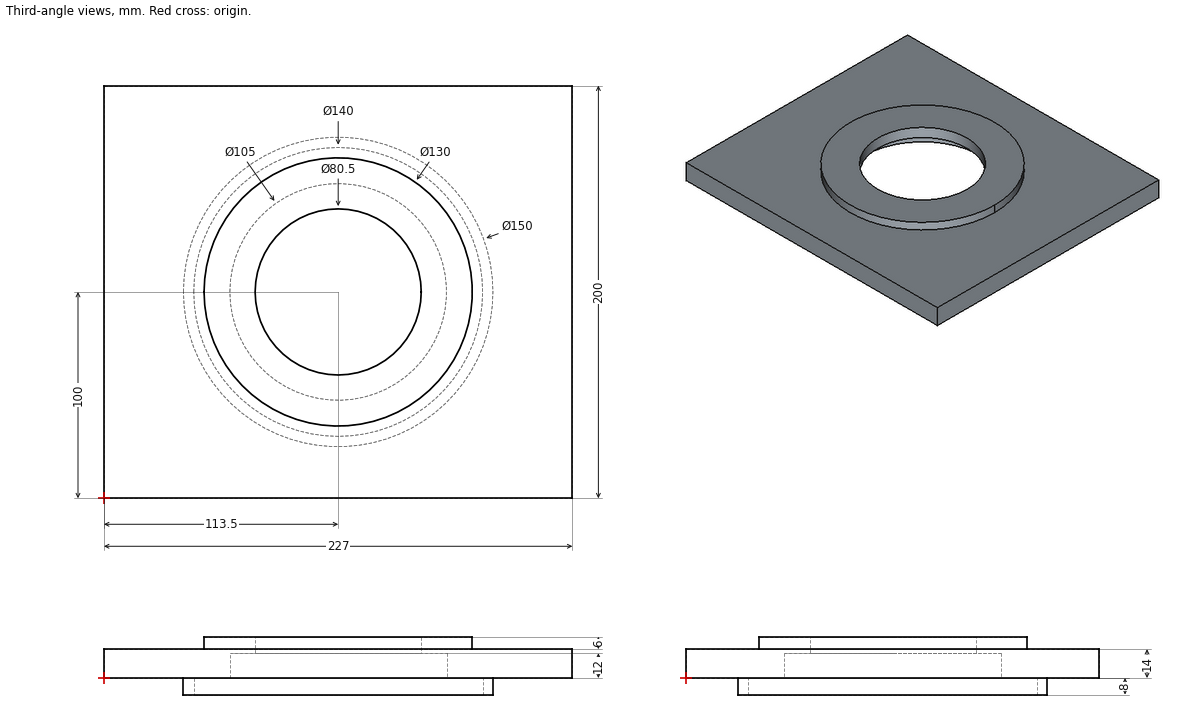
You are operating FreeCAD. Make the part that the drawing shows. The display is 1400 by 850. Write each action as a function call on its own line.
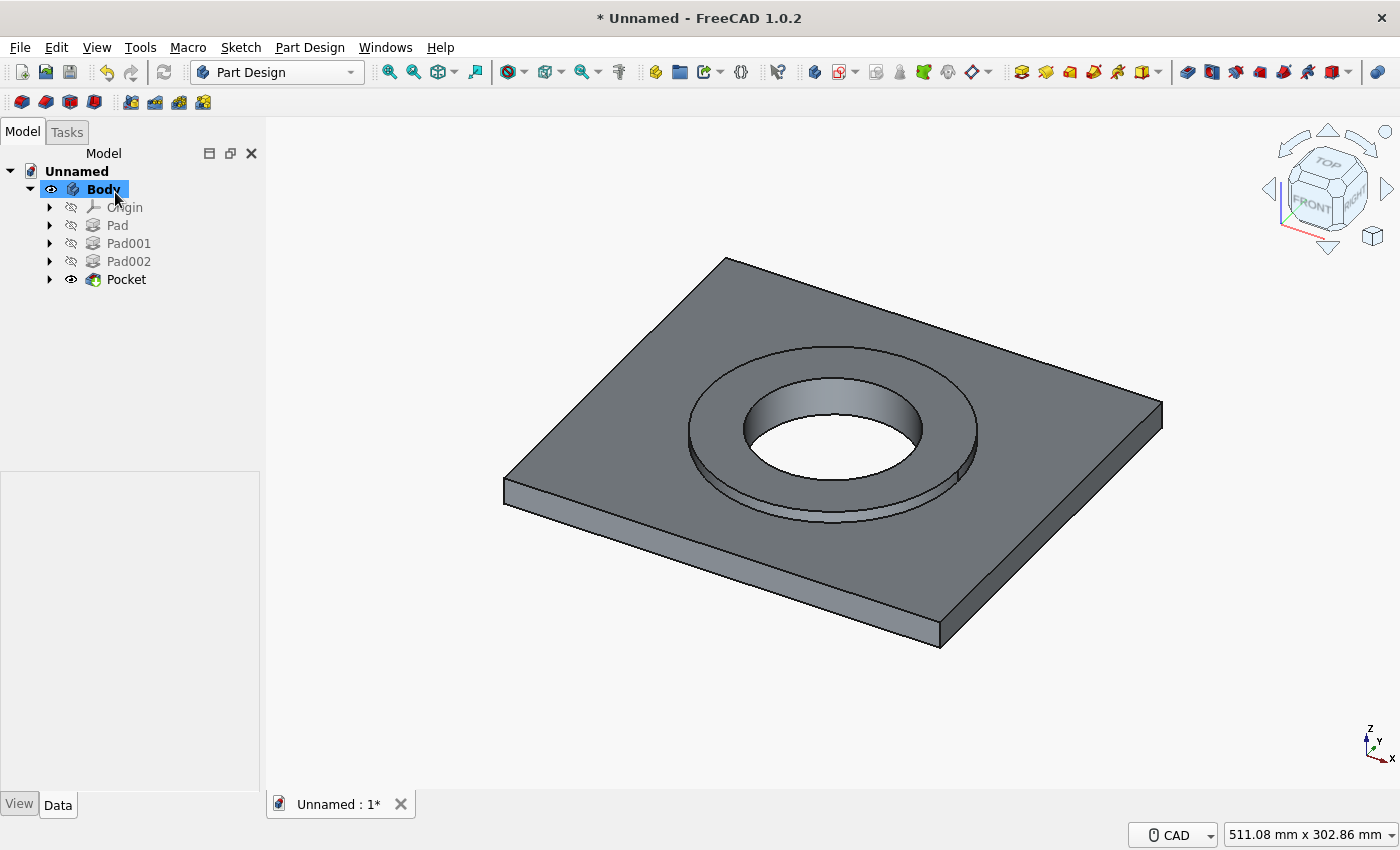
click(840, 72)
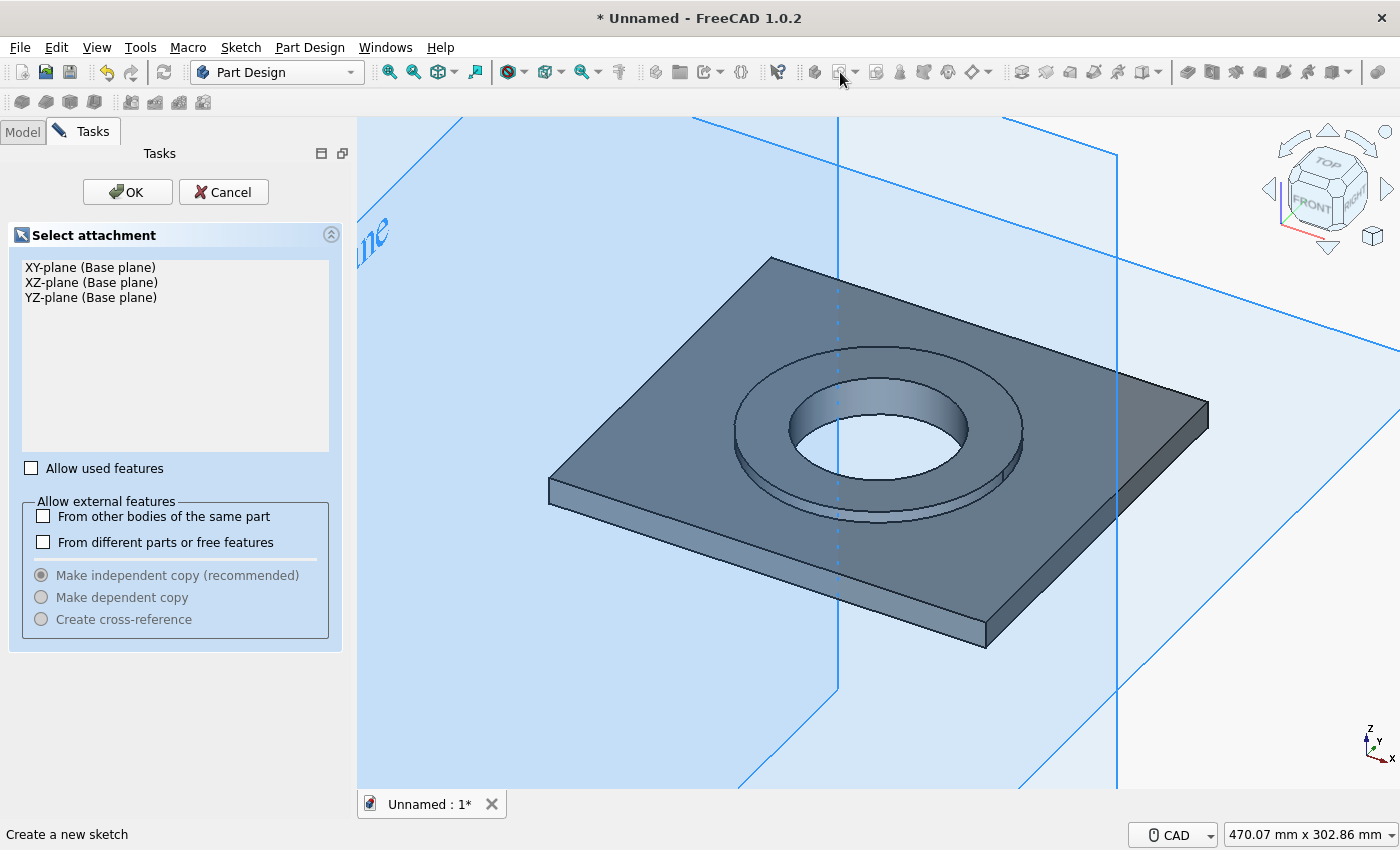
click(82, 268)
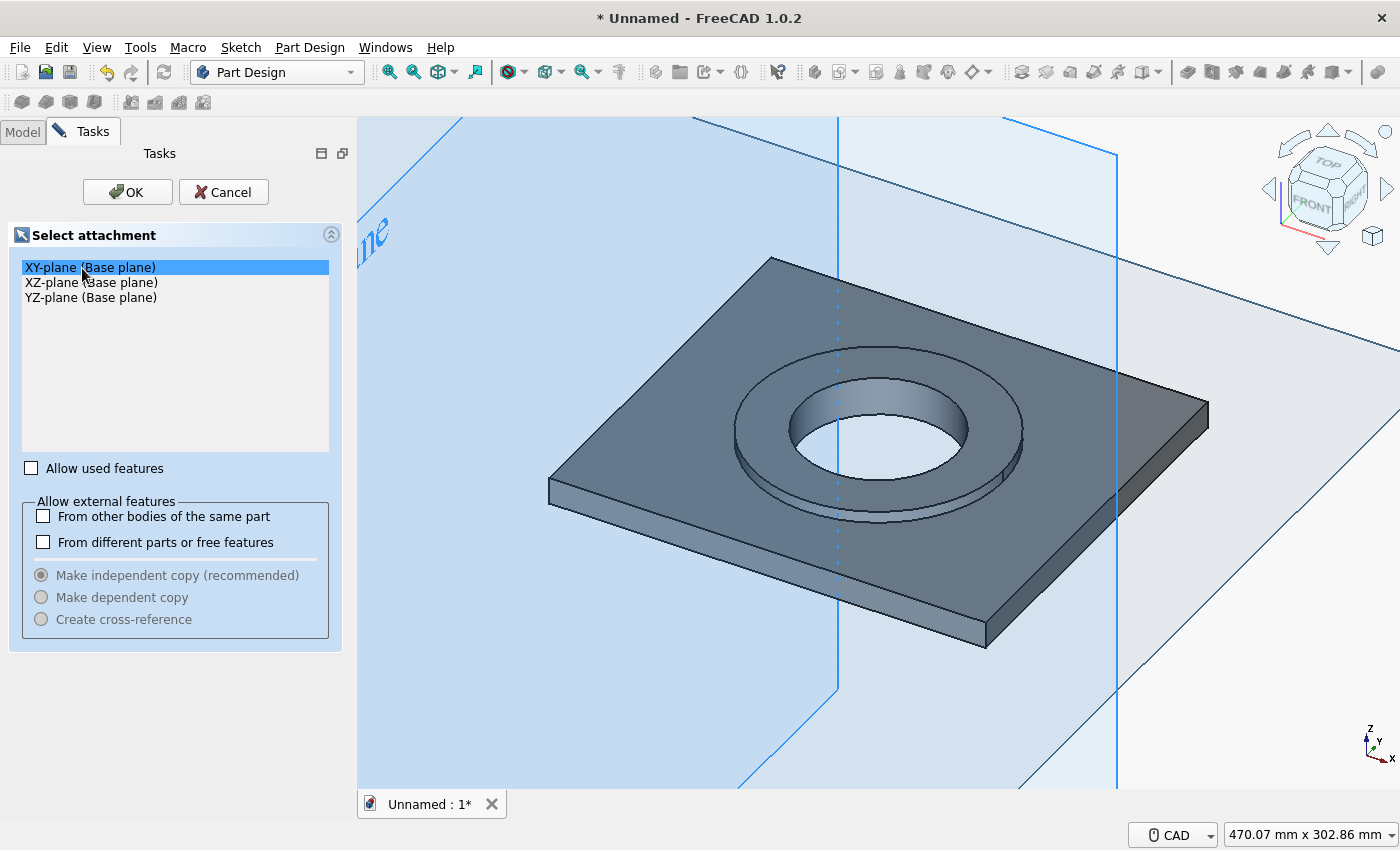
click(128, 192)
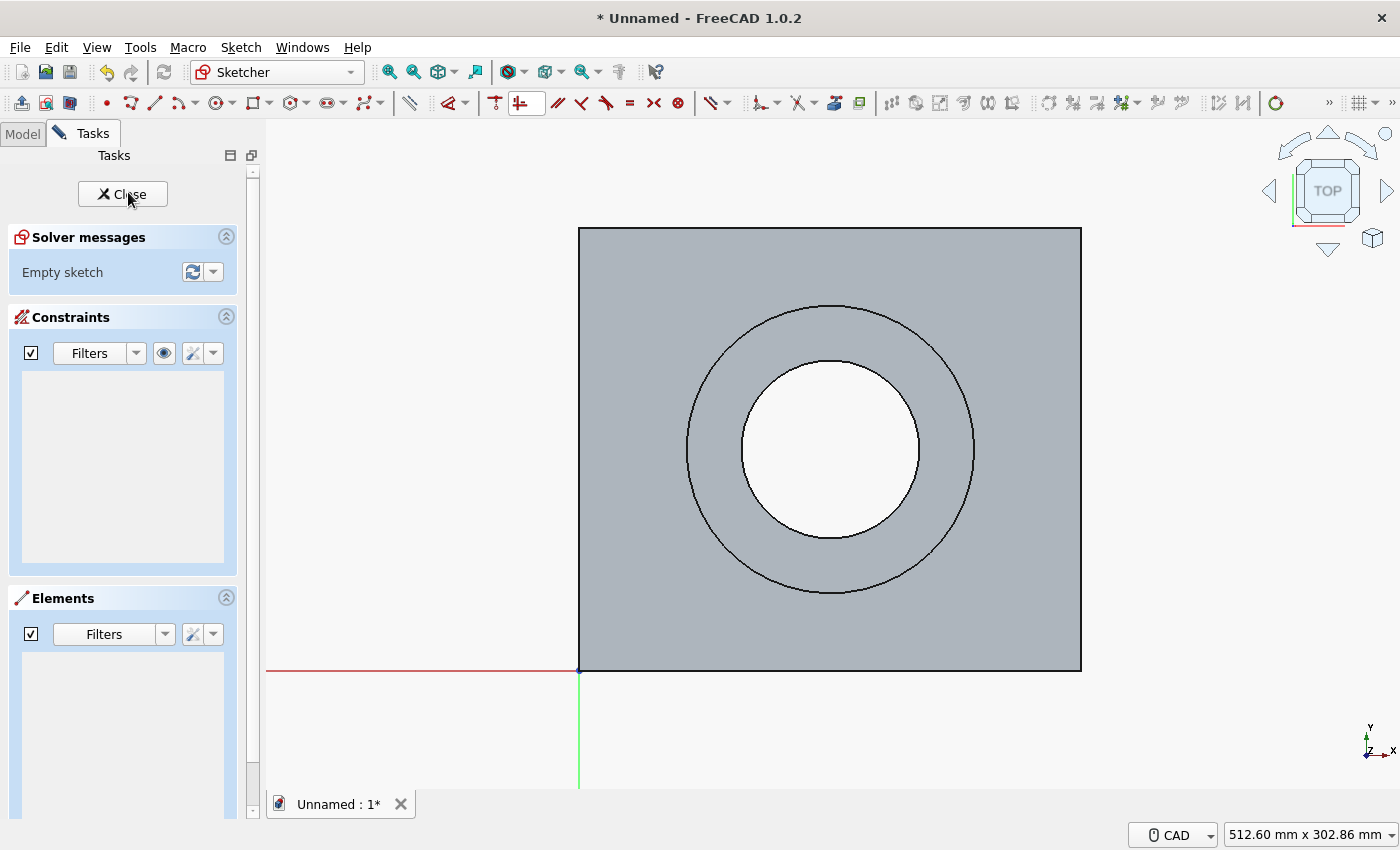
key(q)
key(s)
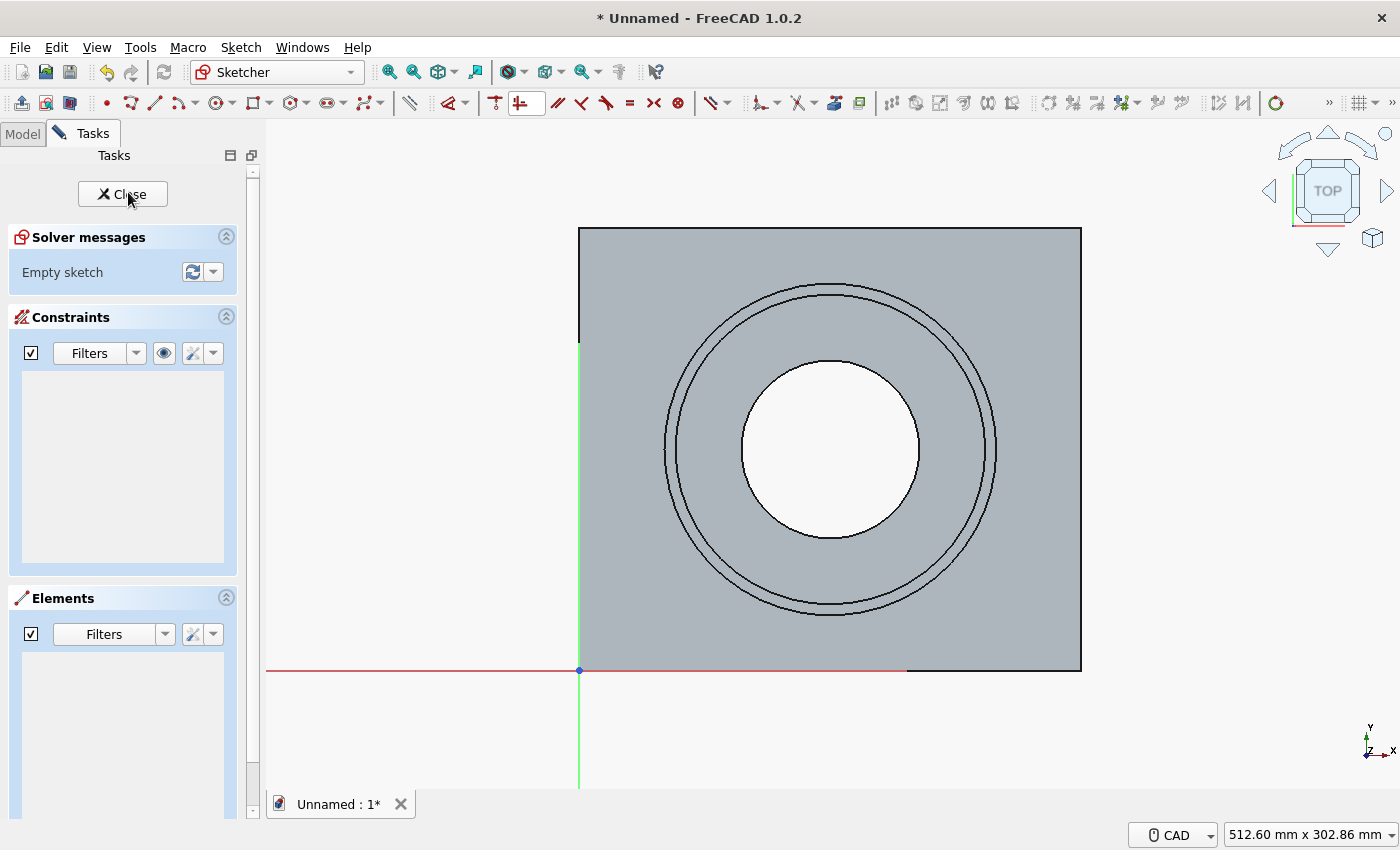
key(g)
key(c)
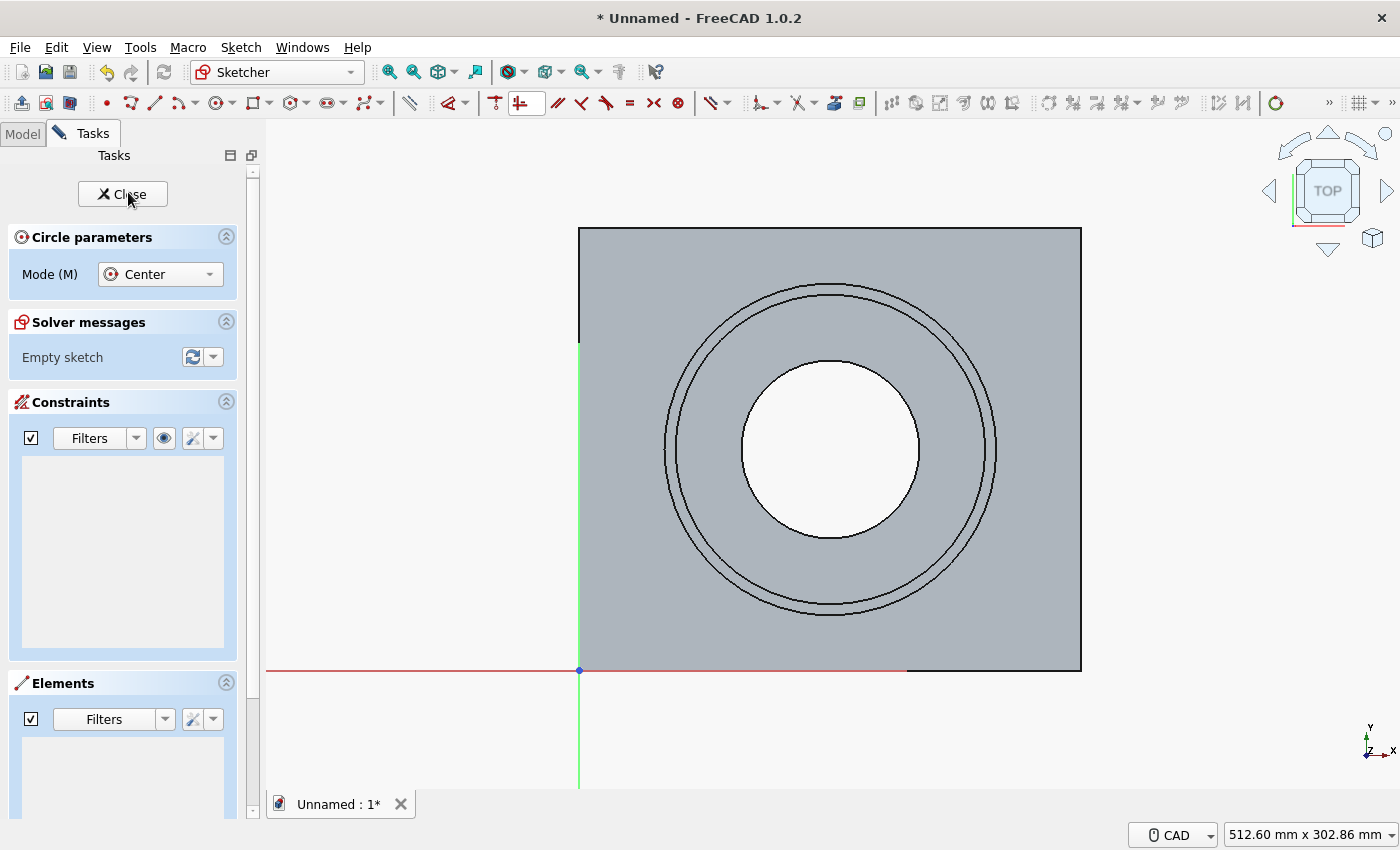
click(830, 449)
click(913, 367)
key(Escape)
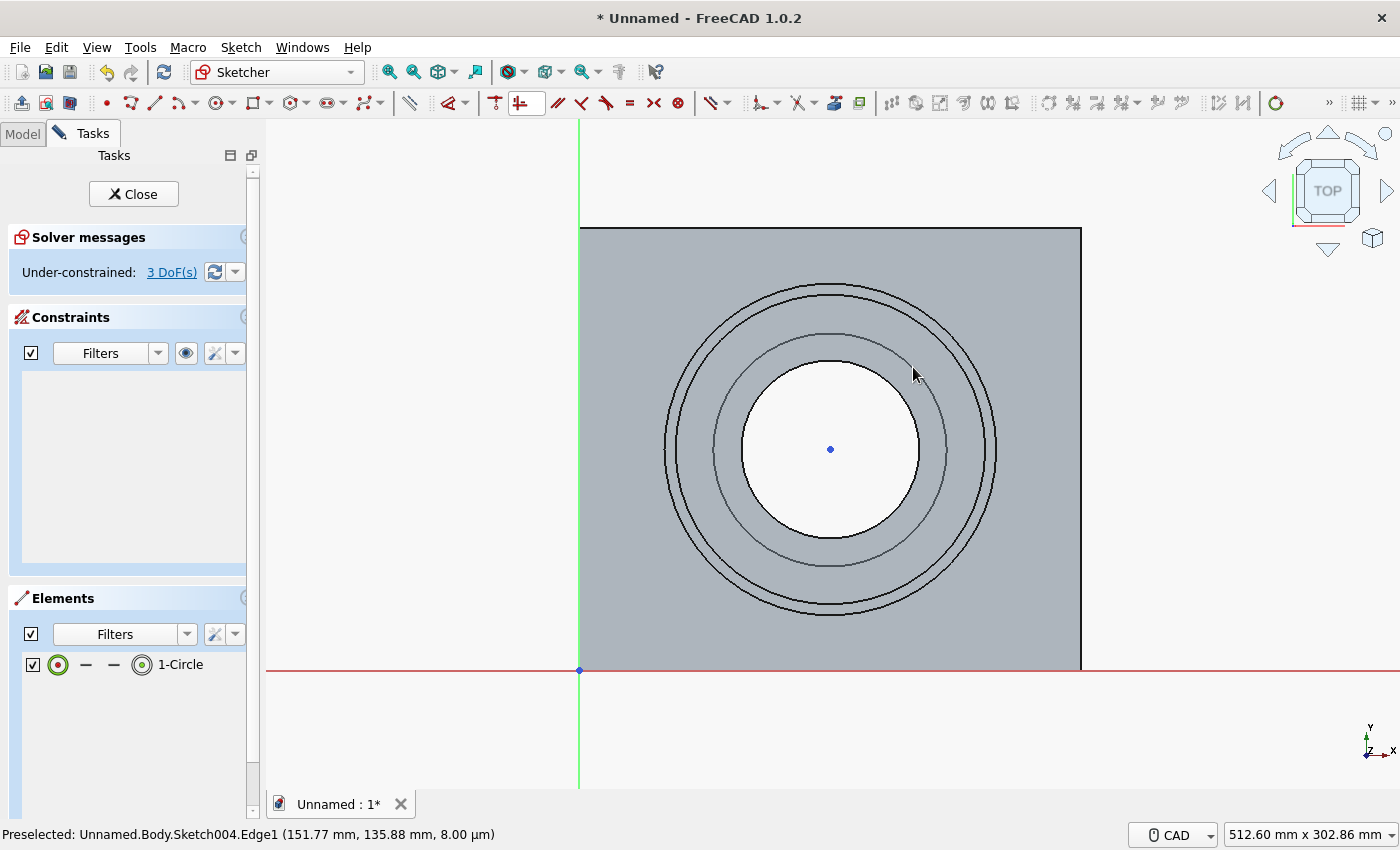
key(d)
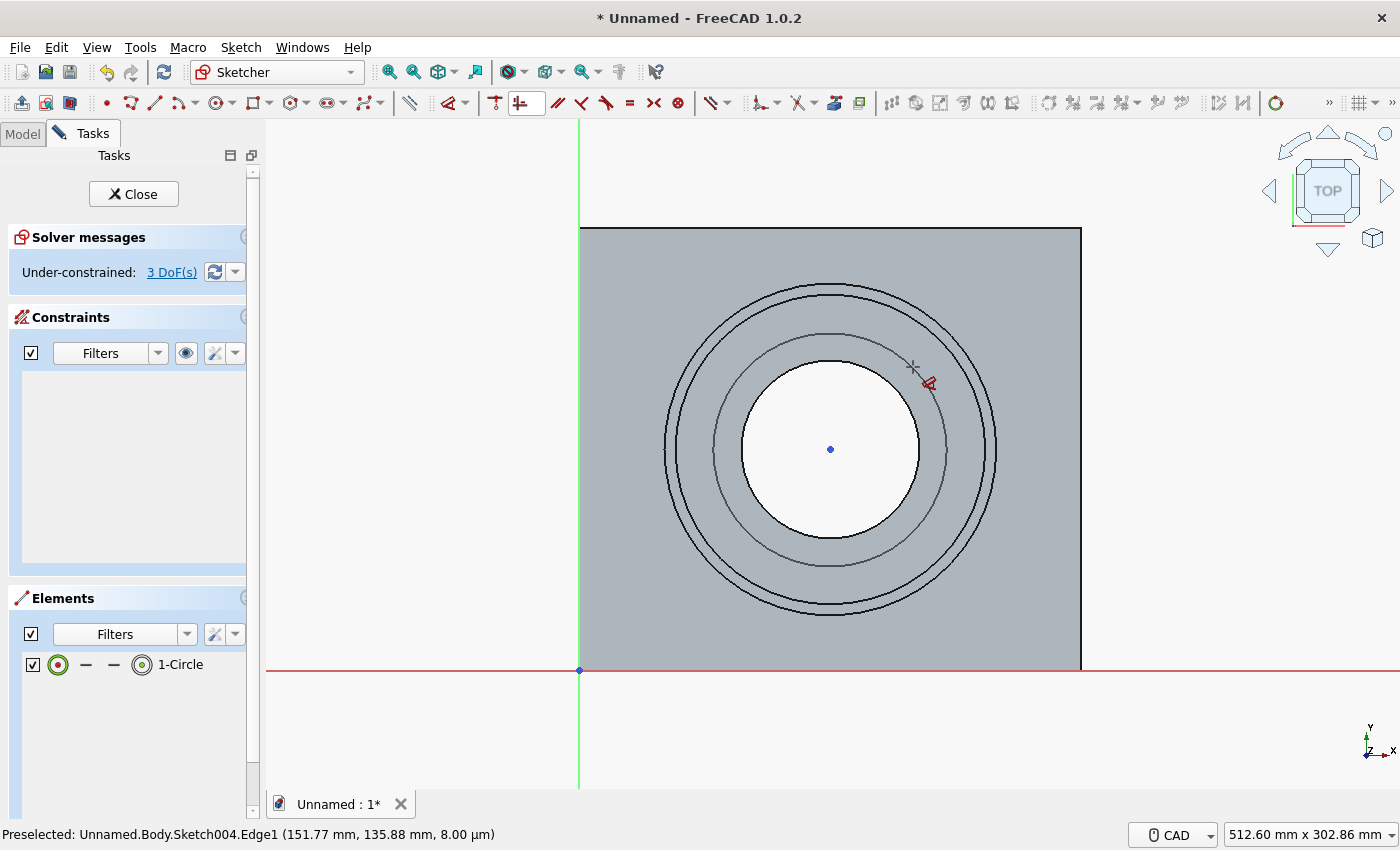
click(912, 367)
click(934, 344)